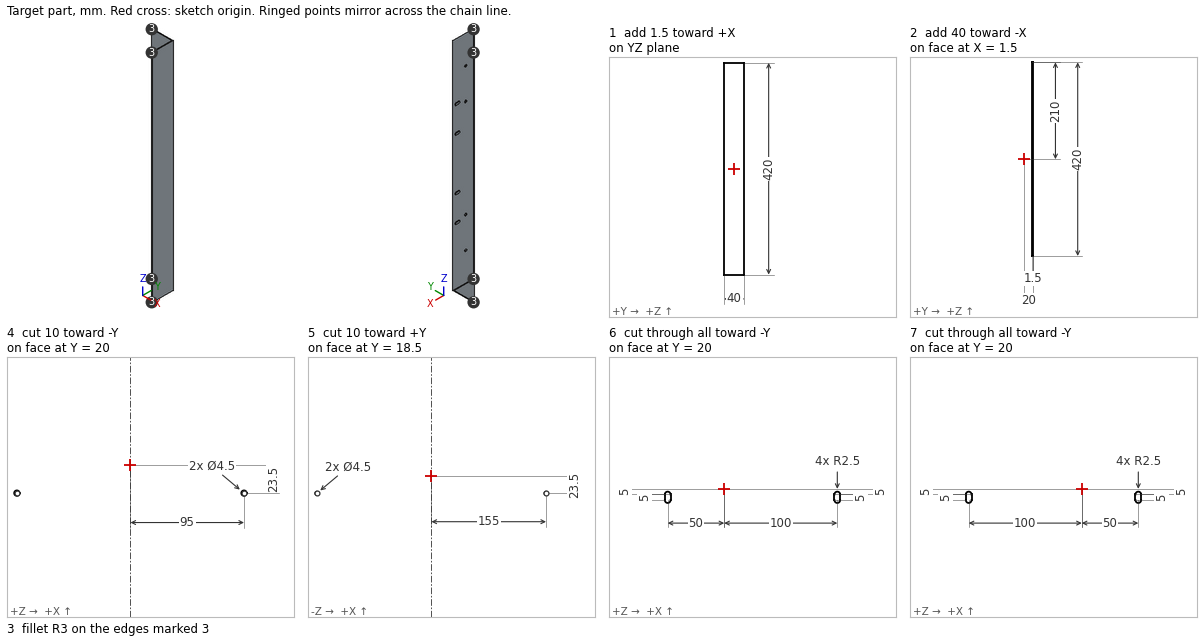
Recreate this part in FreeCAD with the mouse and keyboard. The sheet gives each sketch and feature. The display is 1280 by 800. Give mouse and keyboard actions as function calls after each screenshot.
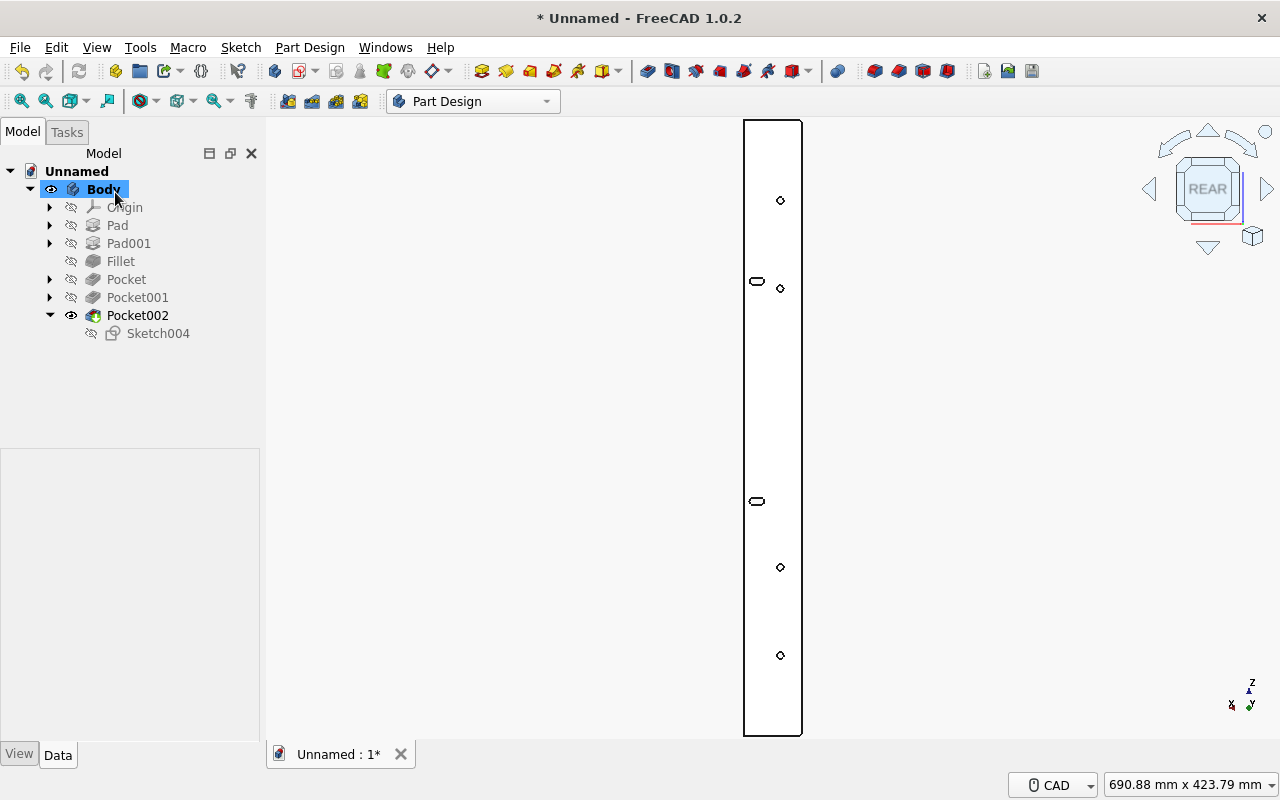
click(773, 603)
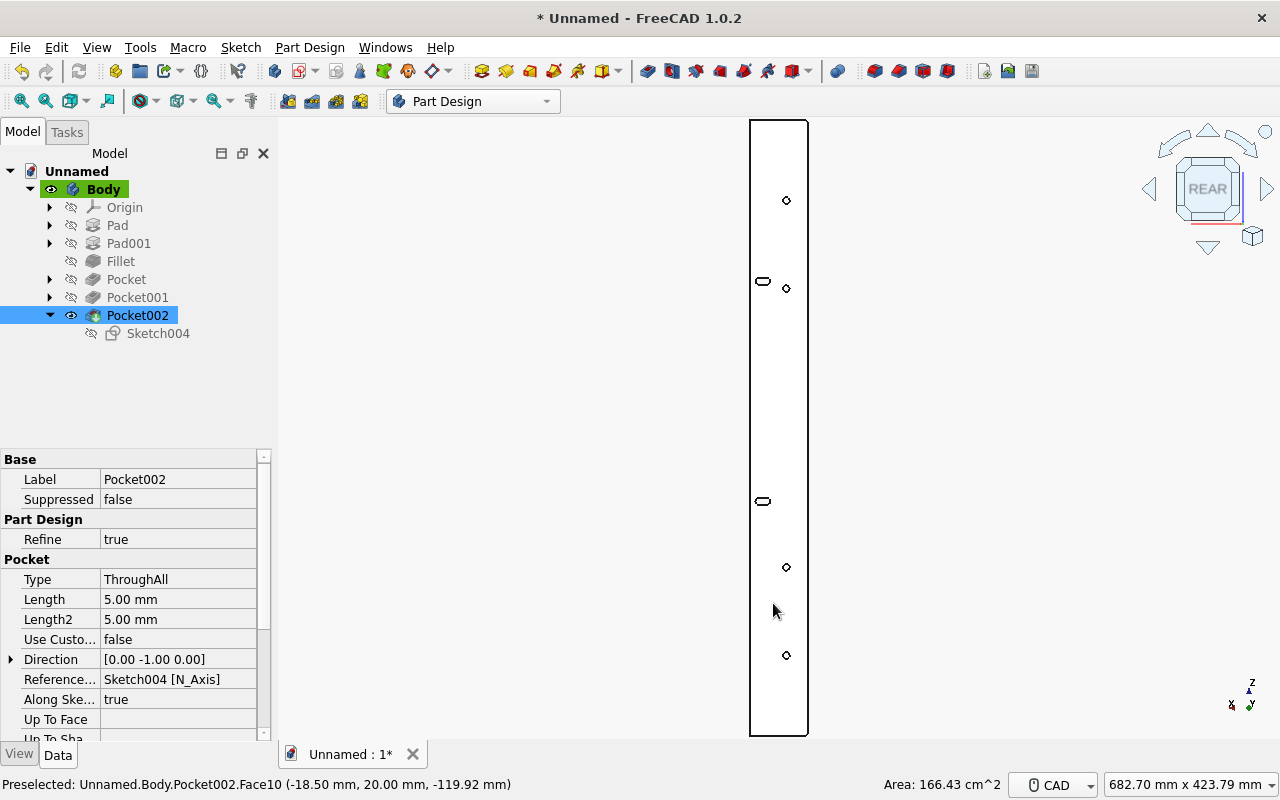
click(300, 72)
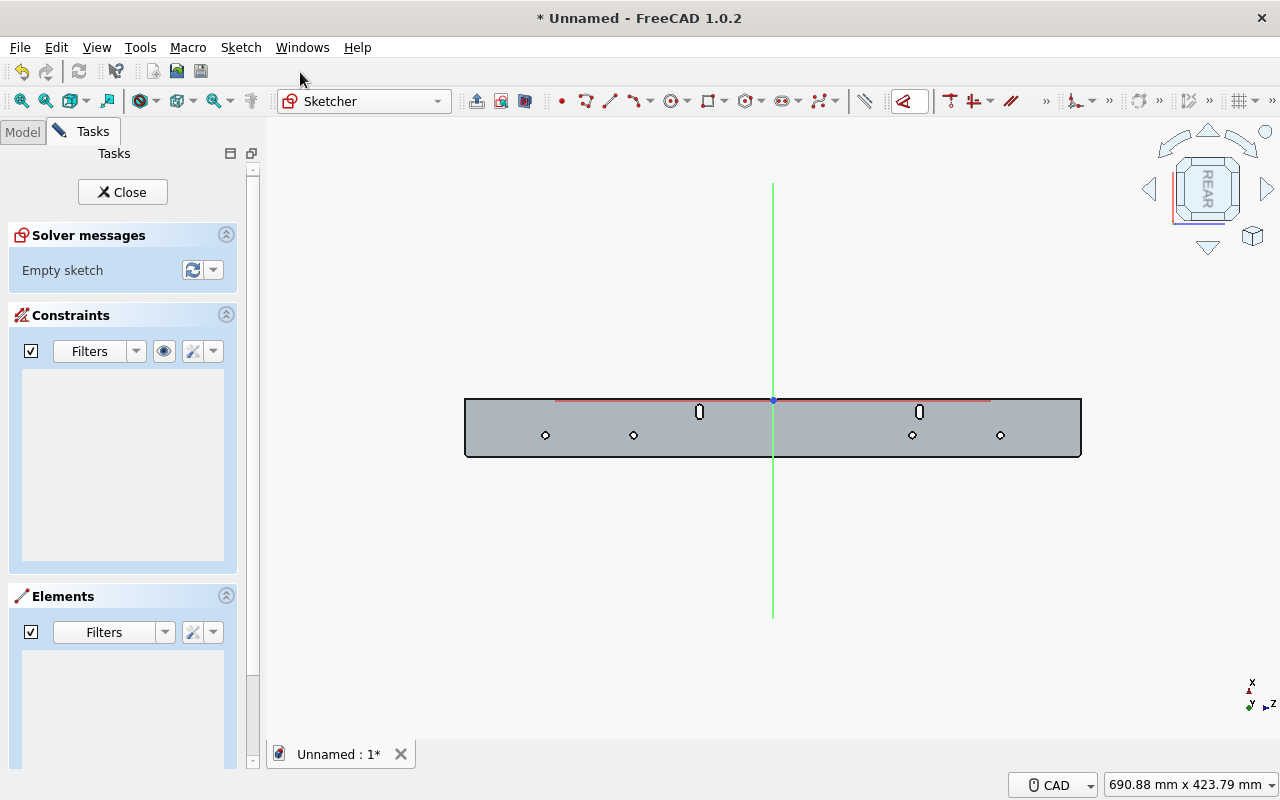
scroll(755, 400, up, 5)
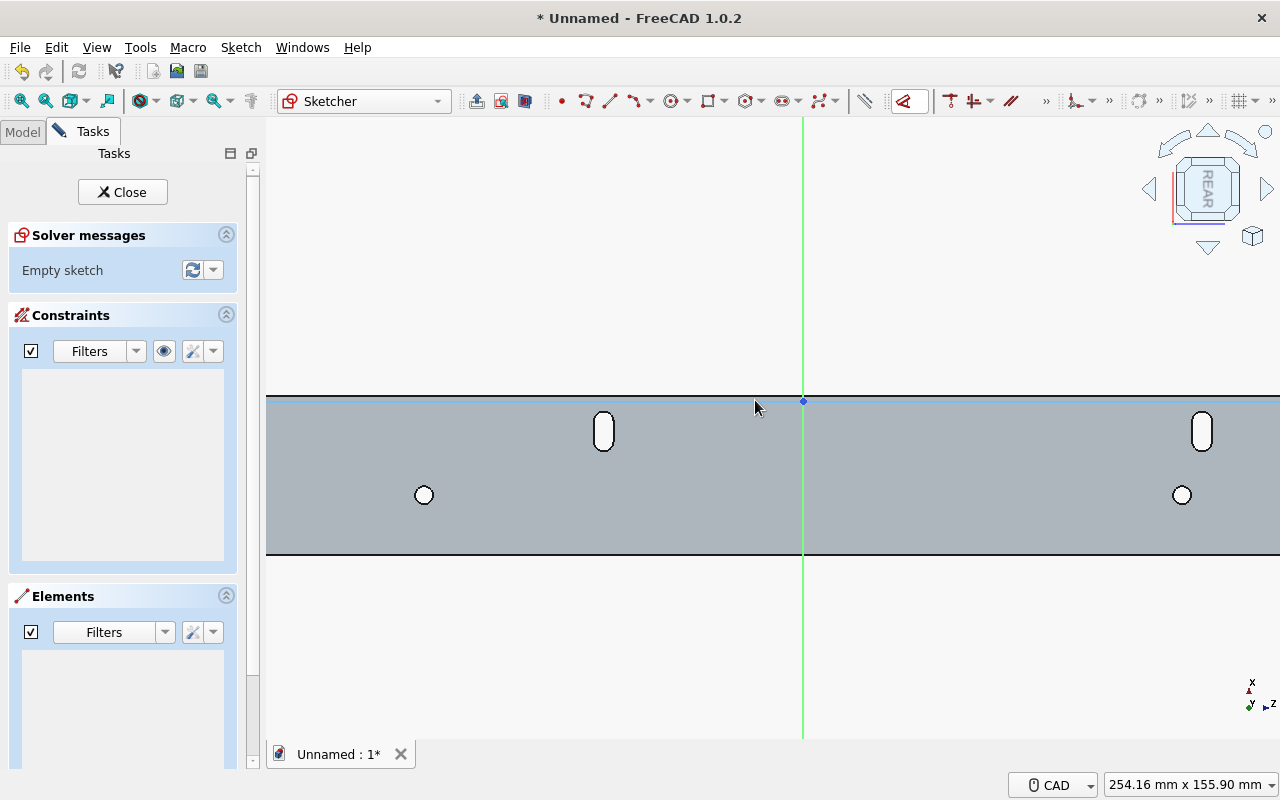
click(782, 102)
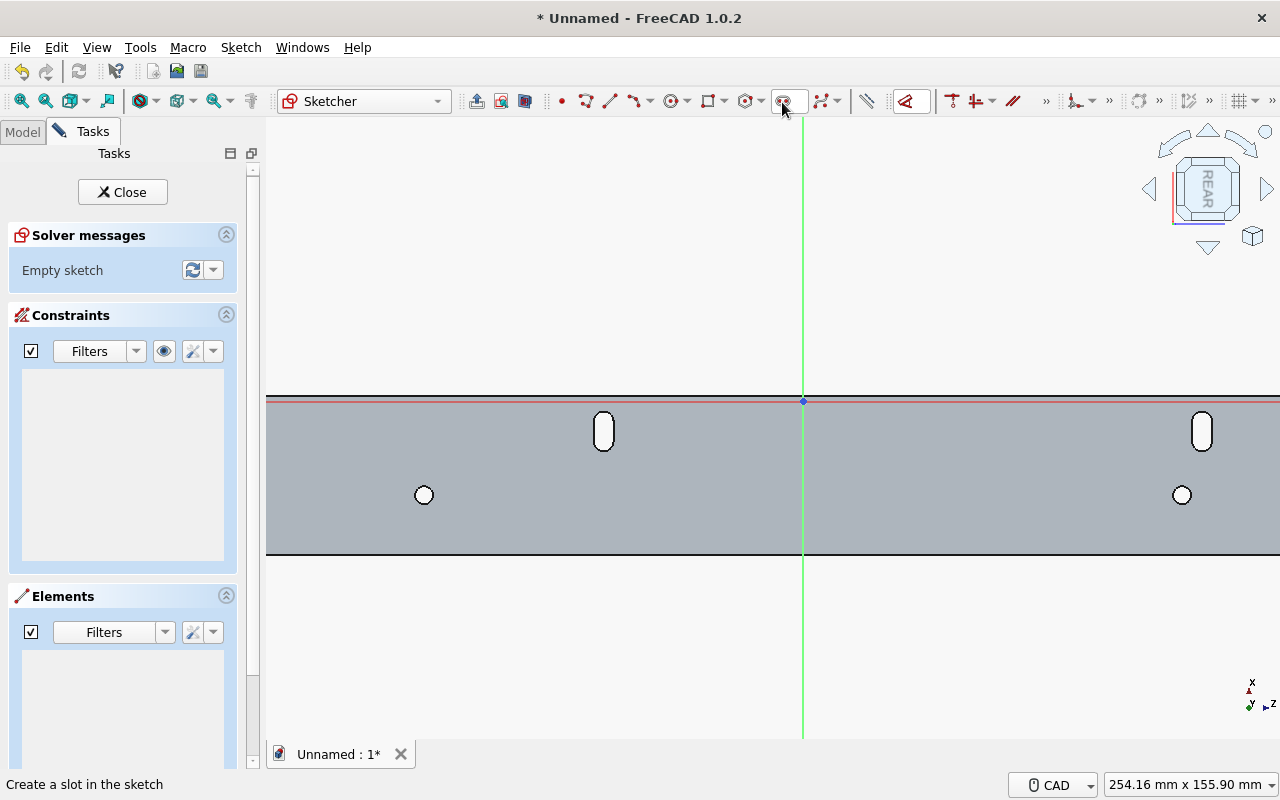
scroll(1003, 441, up, 5)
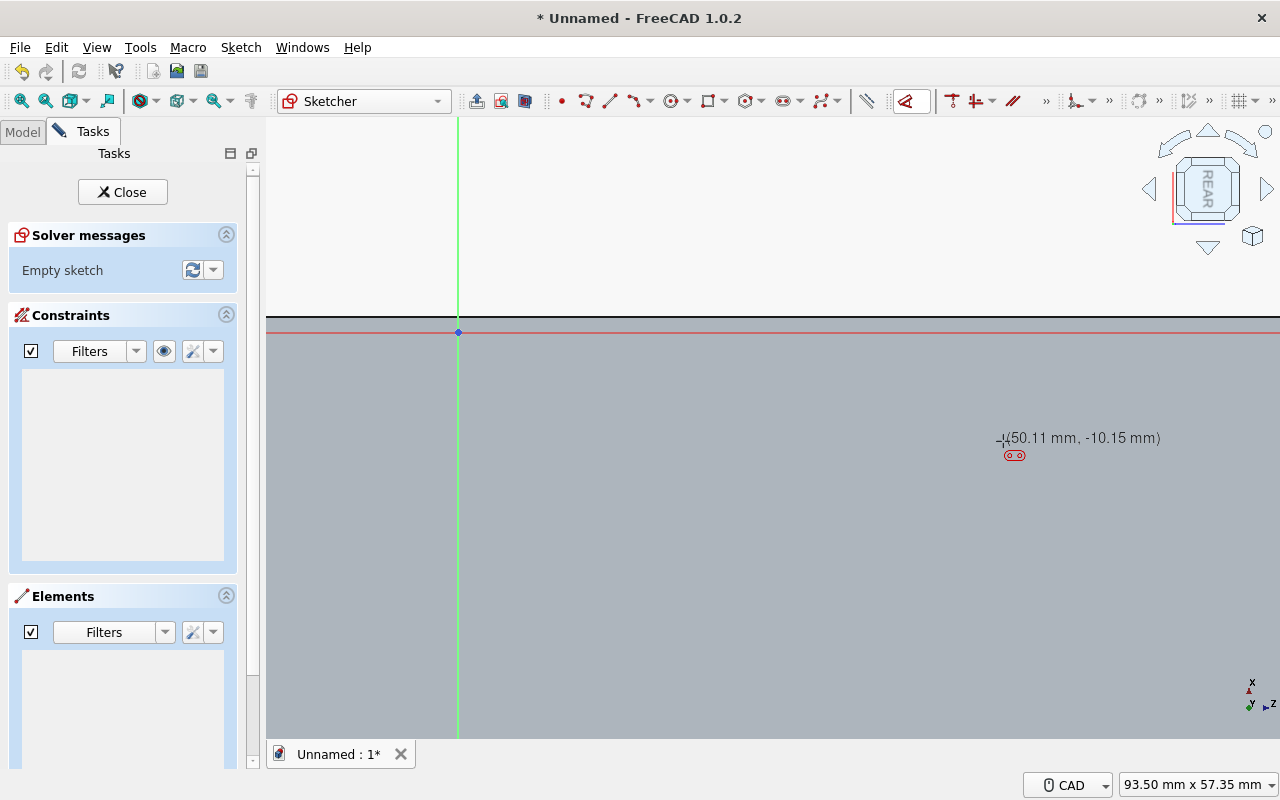
click(1001, 441)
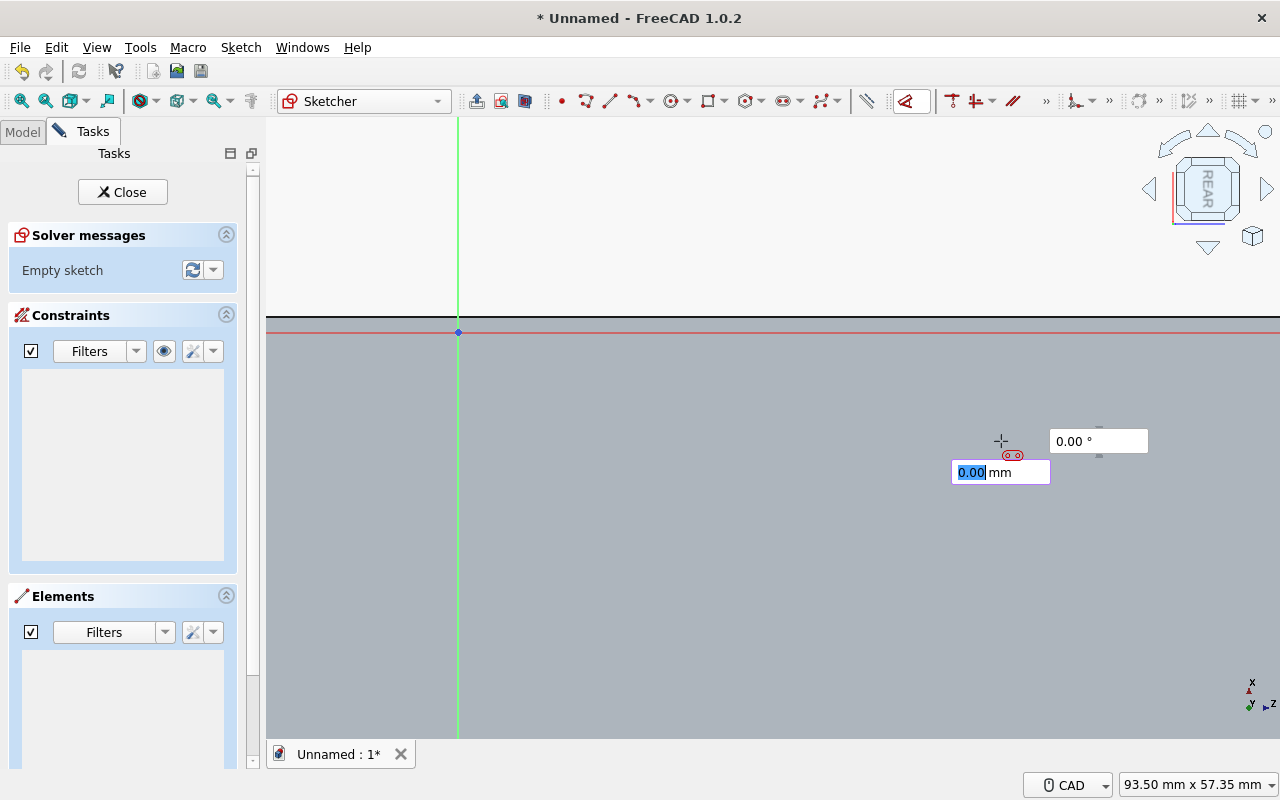
click(1001, 387)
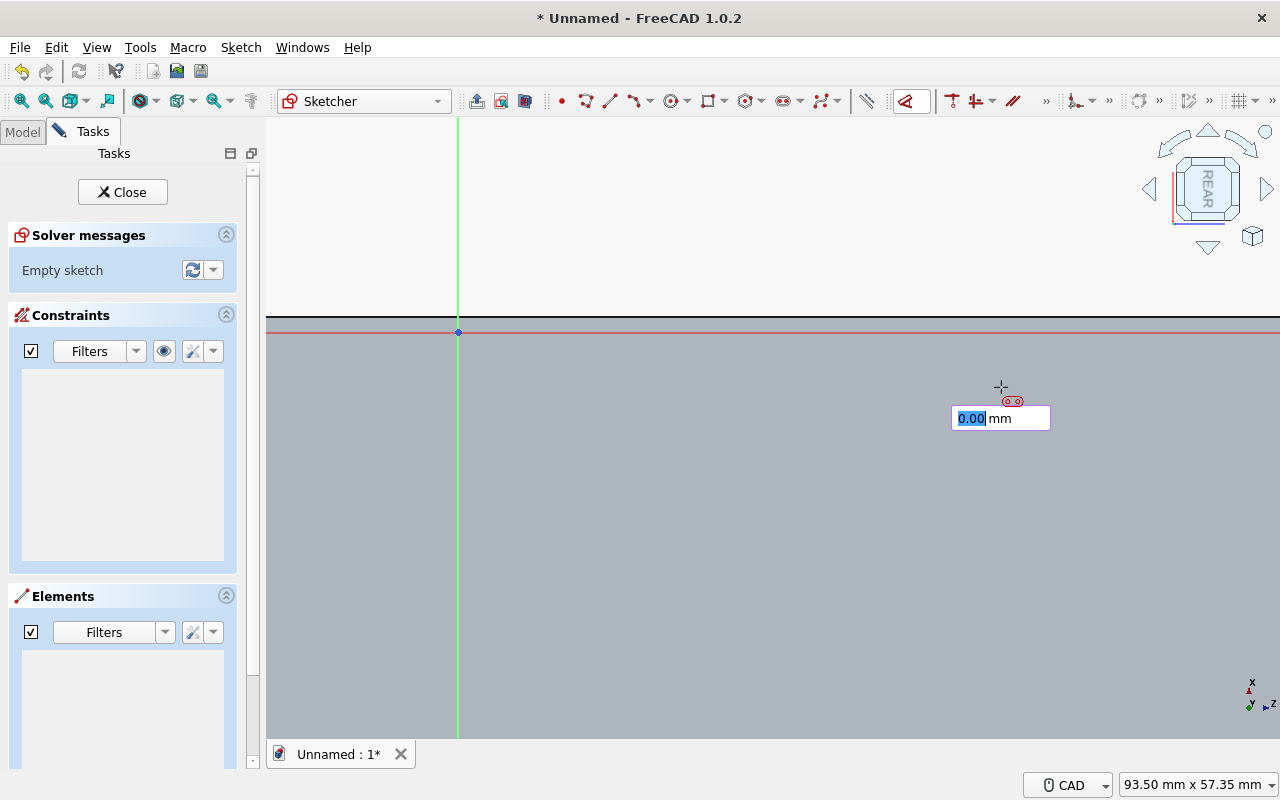
click(1028, 414)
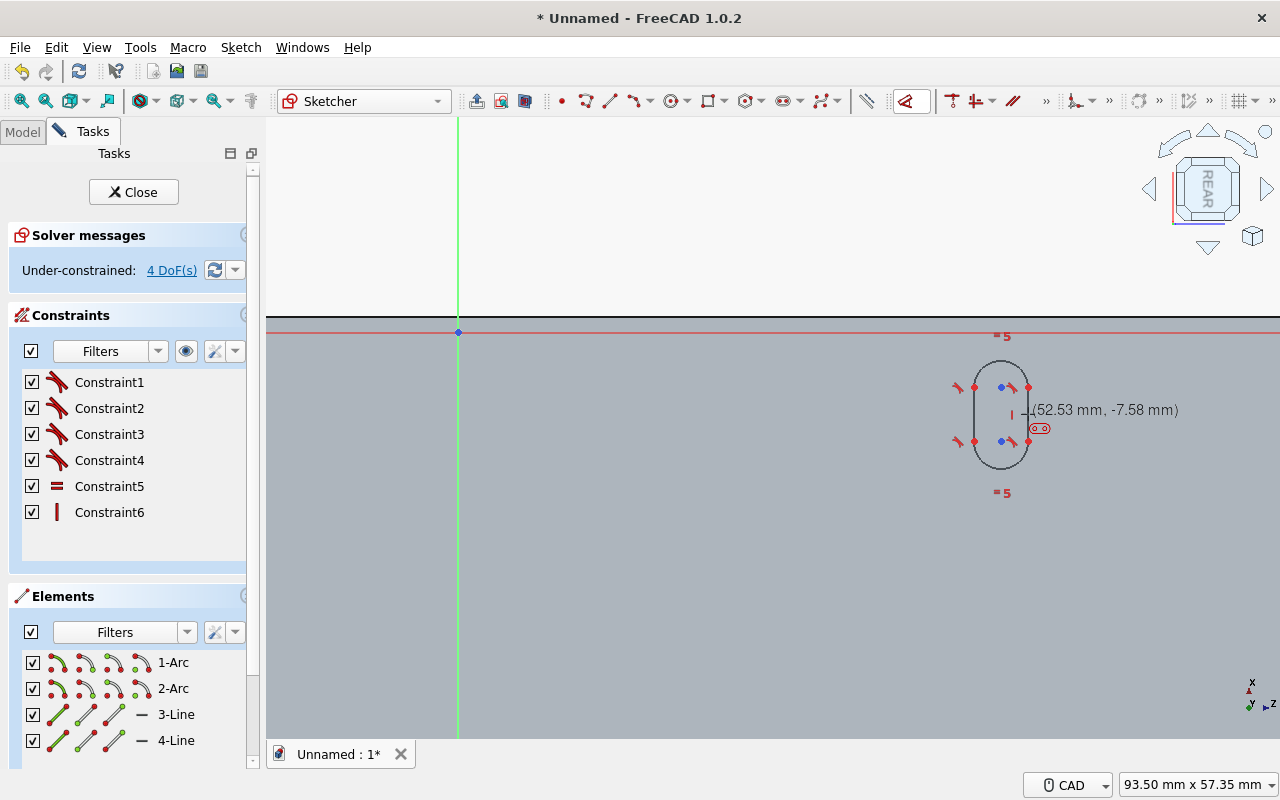
scroll(1006, 444, down, 5)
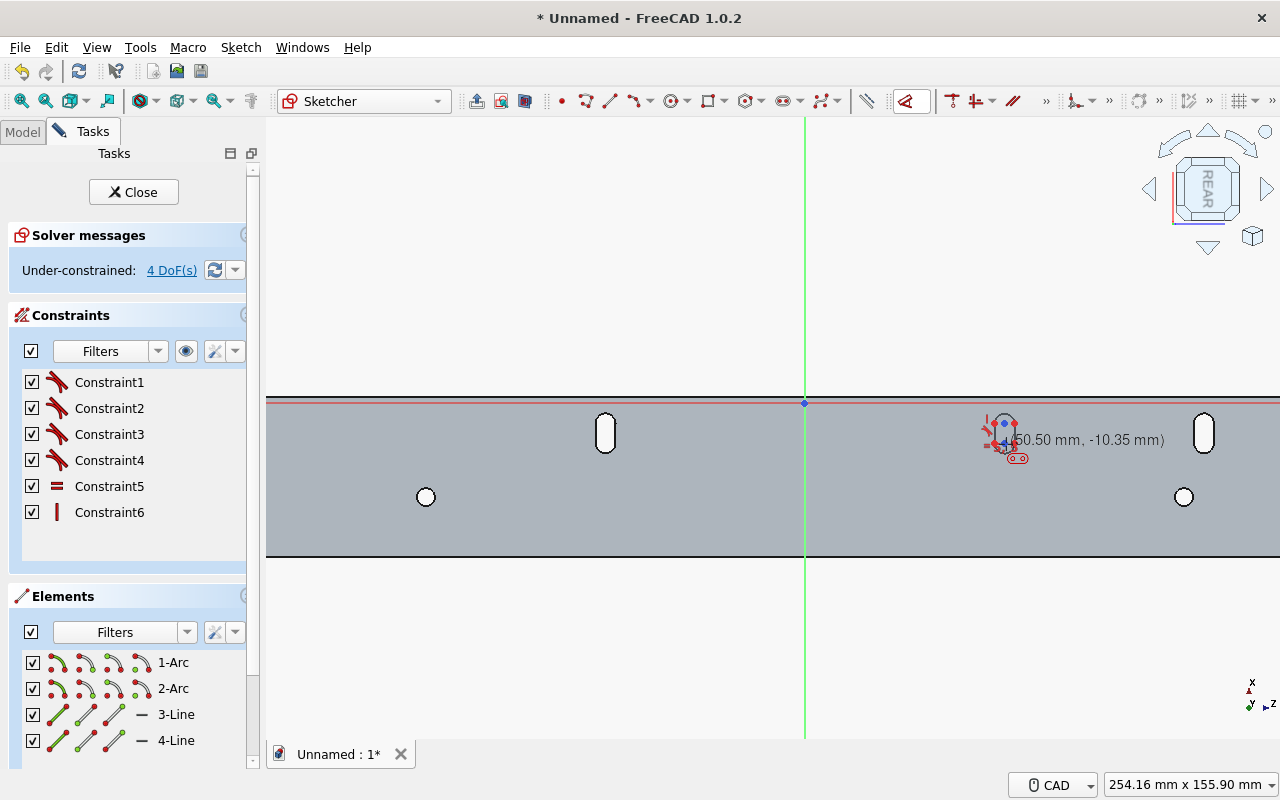
scroll(406, 443, up, 5)